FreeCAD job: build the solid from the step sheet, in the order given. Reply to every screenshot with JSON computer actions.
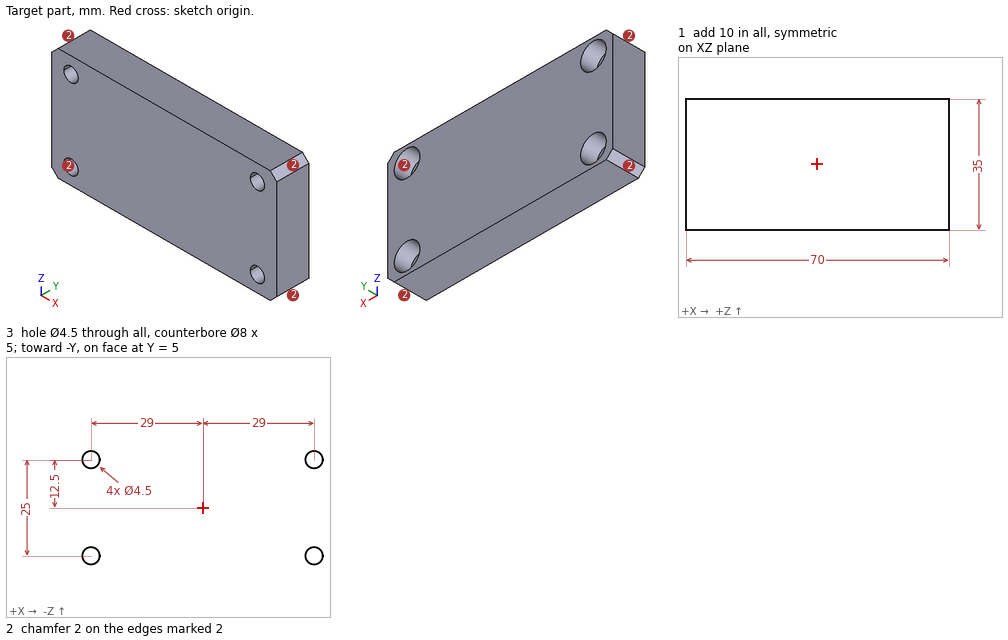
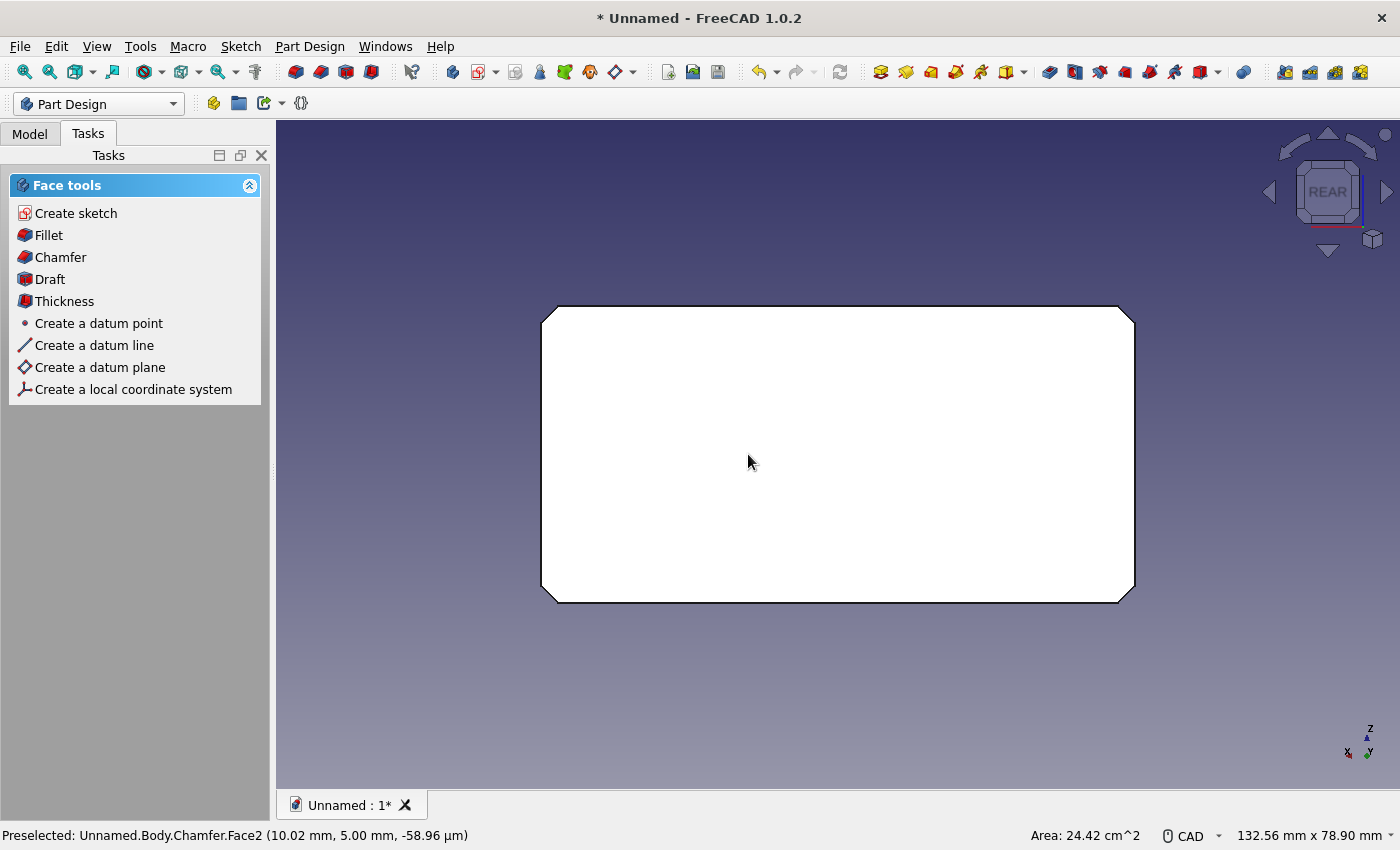
{"action": "left_click", "coordinate": [478, 72]}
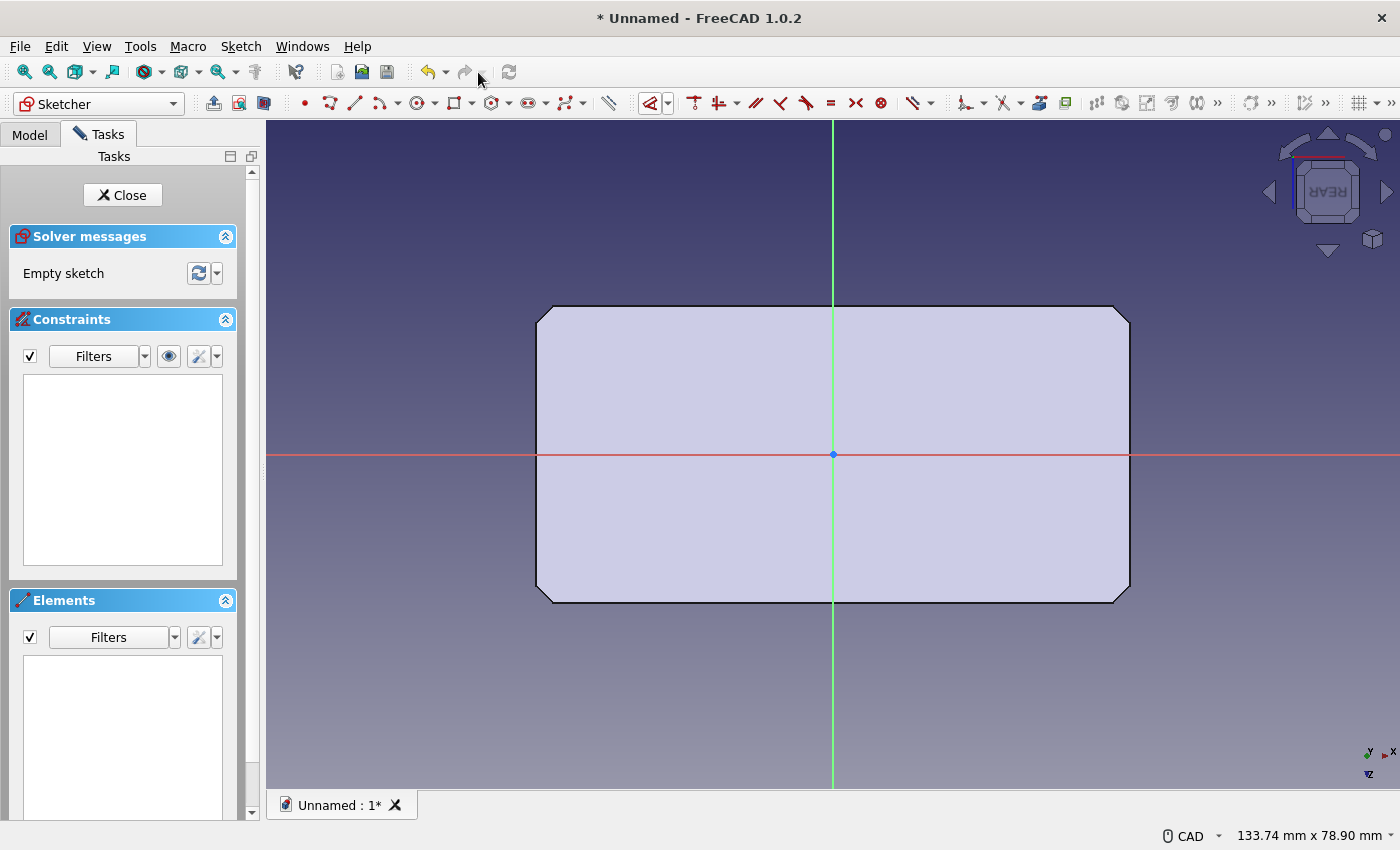
{"action": "left_click", "coordinate": [416, 104]}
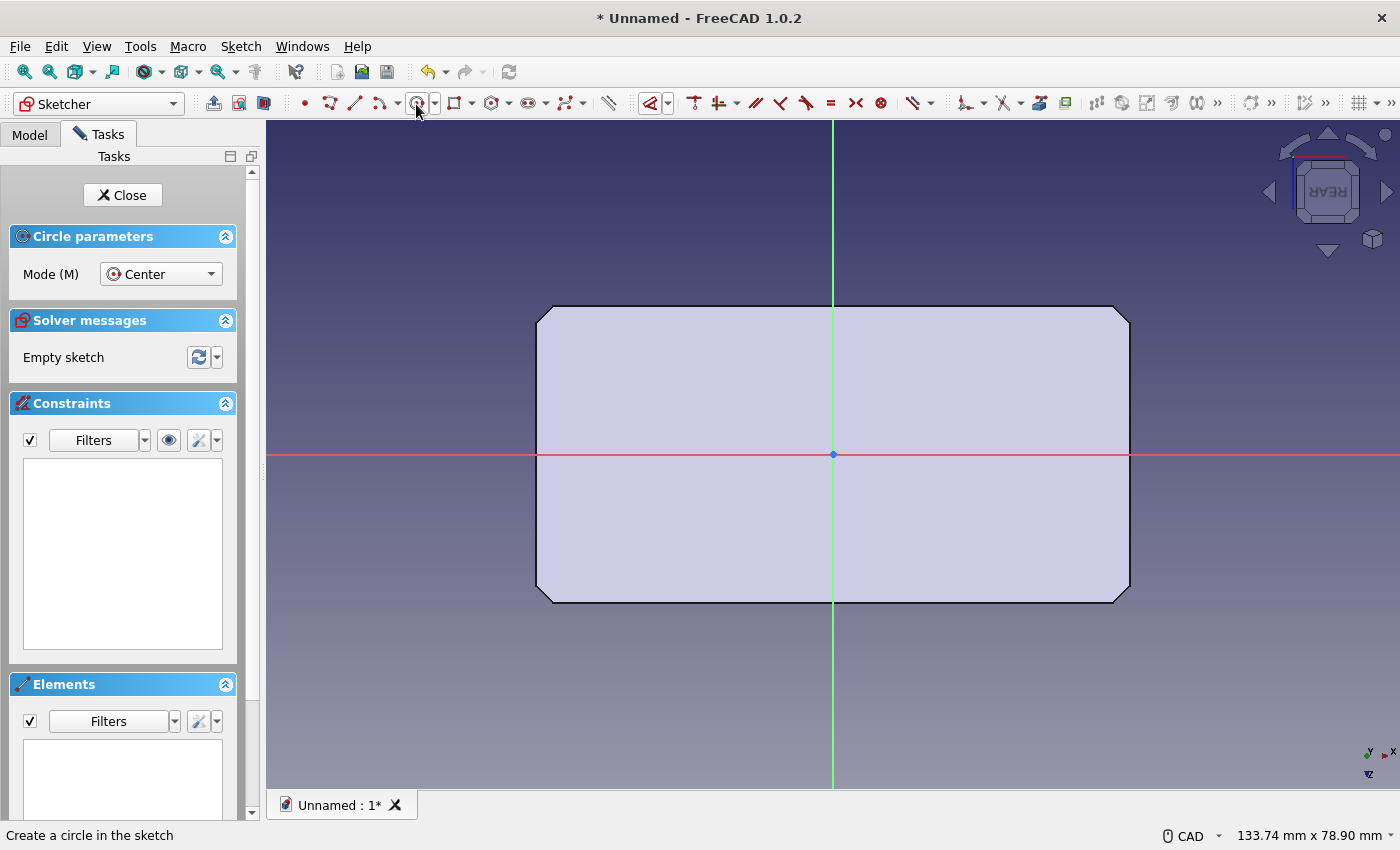
{"action": "left_click", "coordinate": [587, 349]}
{"action": "left_click", "coordinate": [601, 335]}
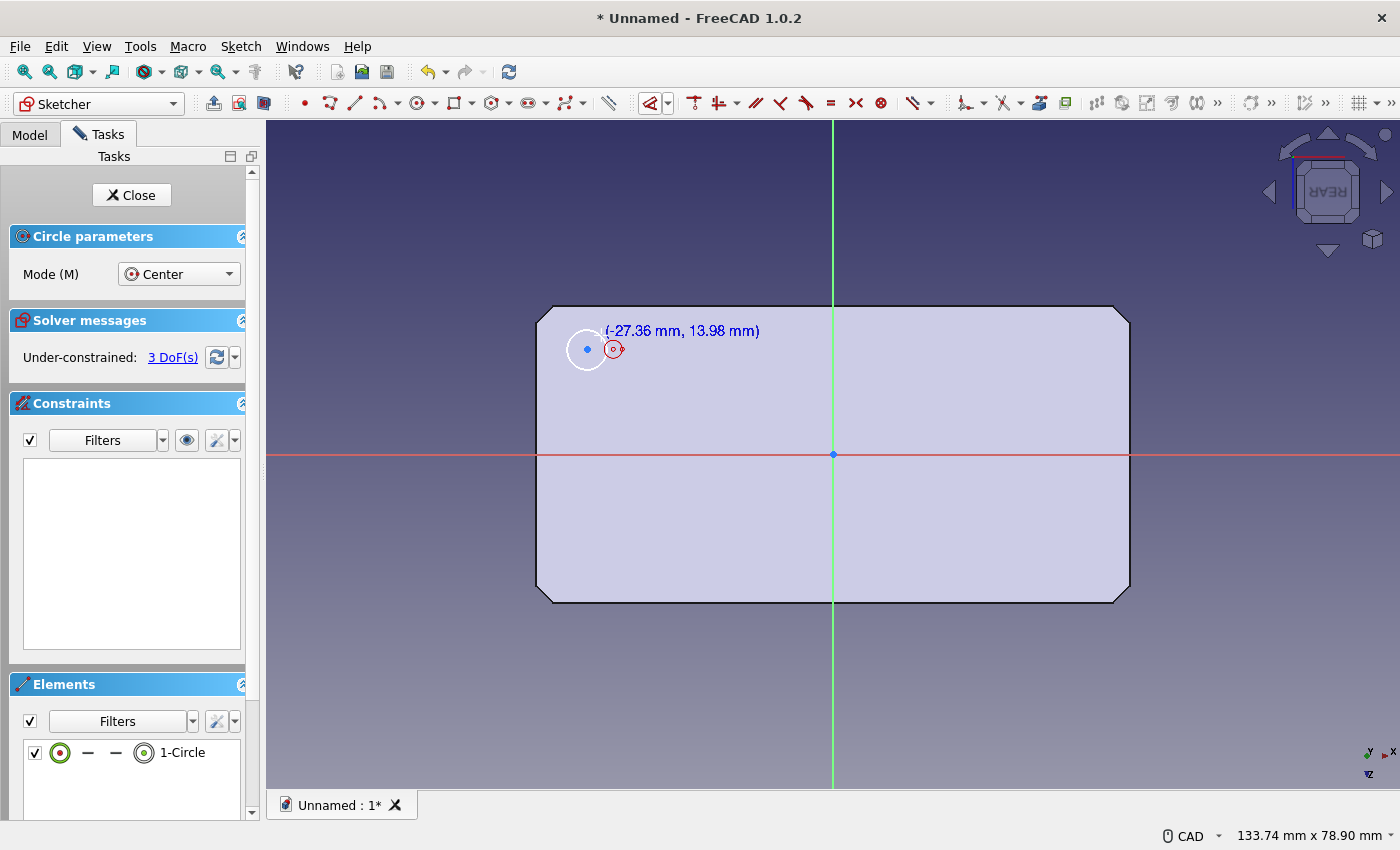
{"action": "left_click", "coordinate": [587, 560]}
{"action": "left_click", "coordinate": [601, 547]}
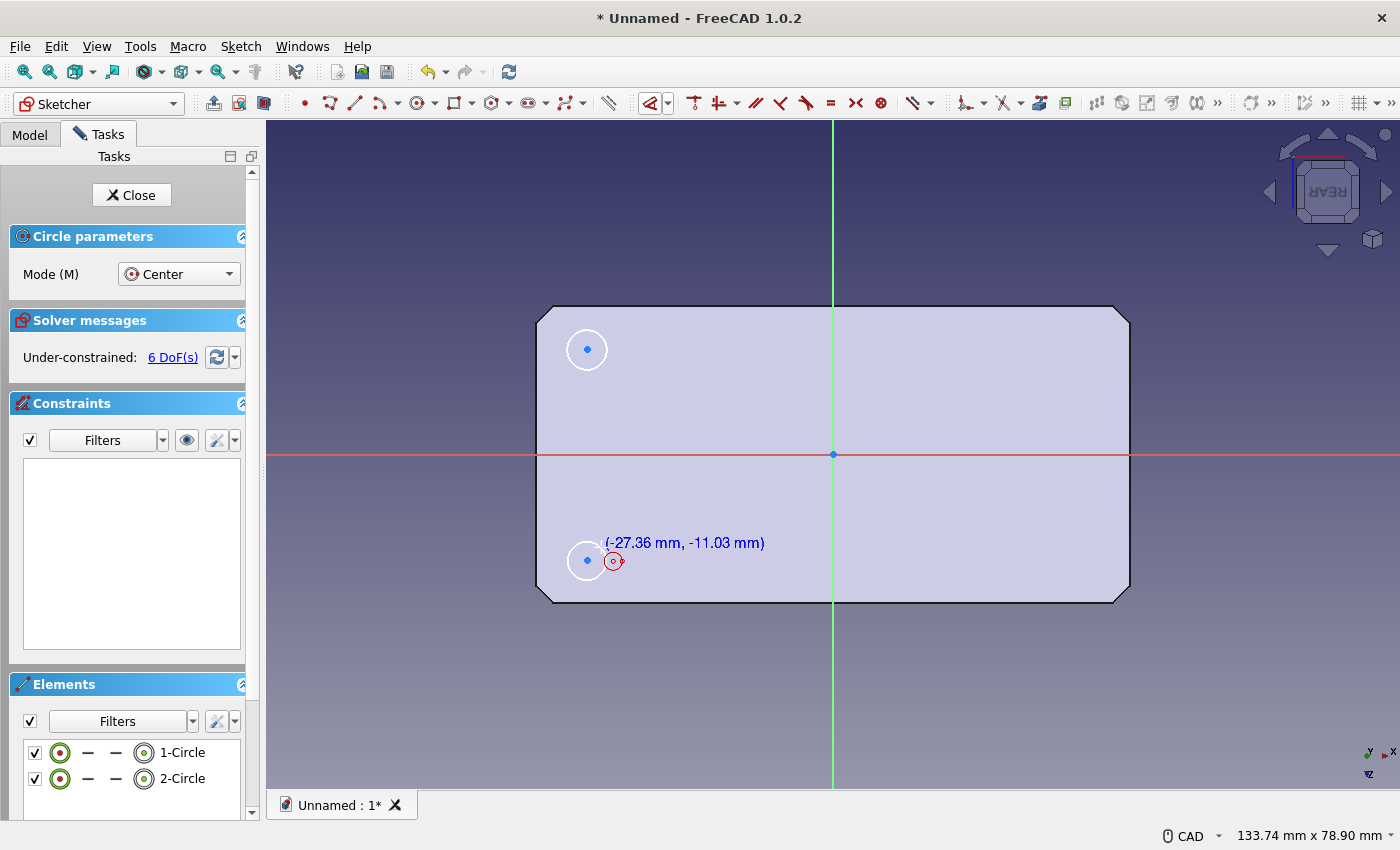
{"action": "left_click", "coordinate": [1079, 349]}
{"action": "left_click", "coordinate": [1092, 335]}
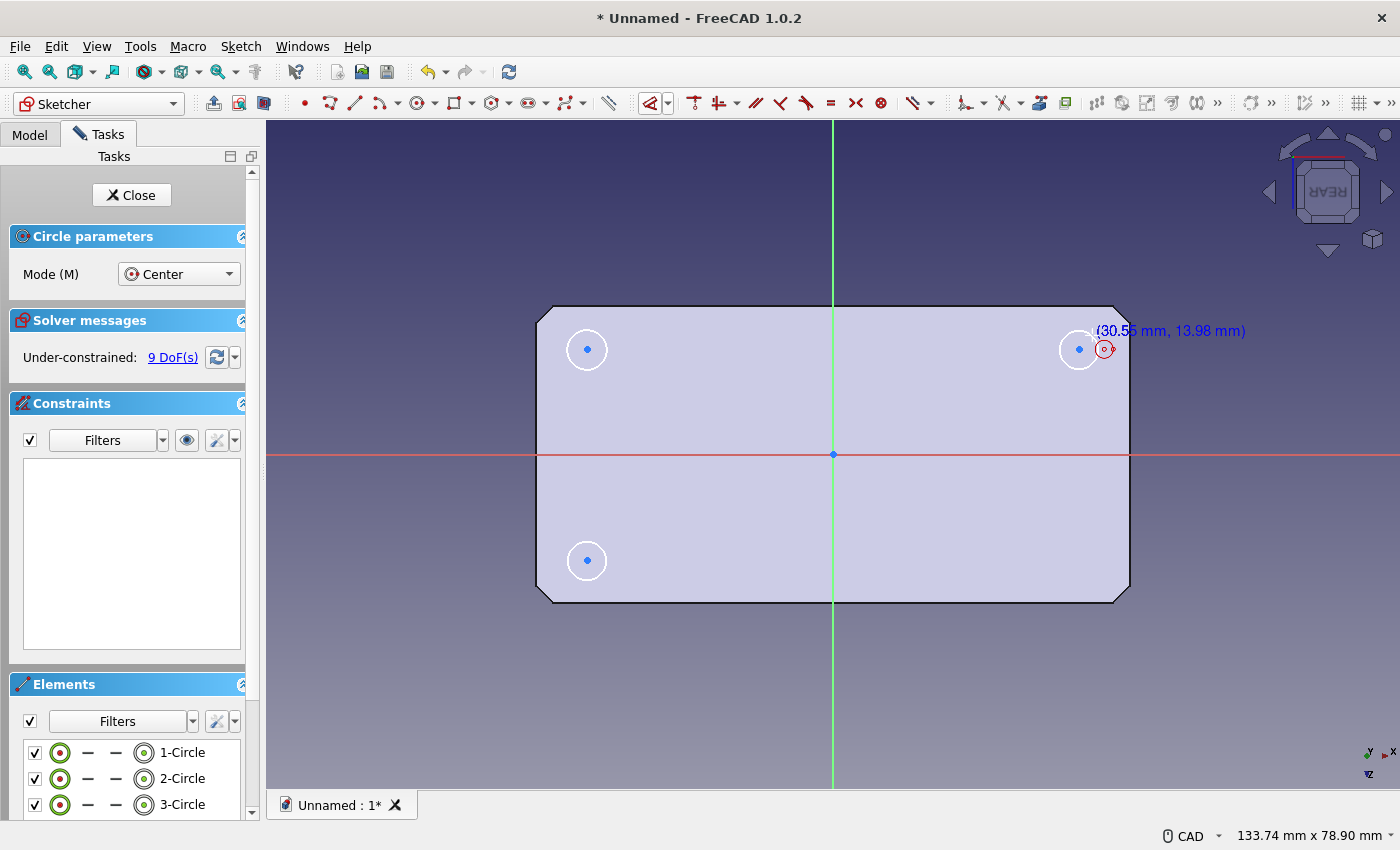
{"action": "left_click", "coordinate": [1079, 560]}
{"action": "left_click", "coordinate": [1092, 547]}
{"action": "key", "text": "Escape"}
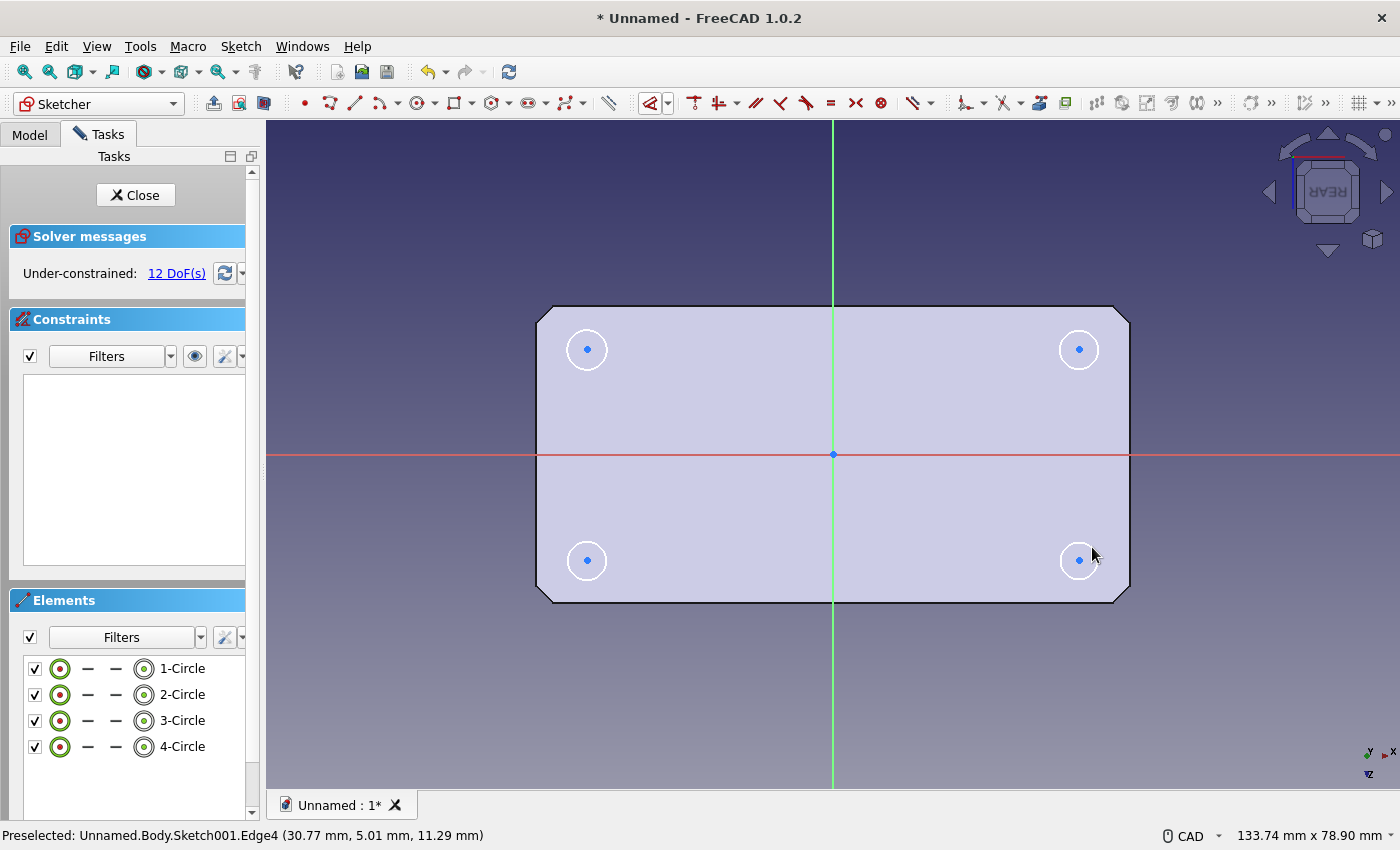
{"action": "left_click", "coordinate": [601, 336]}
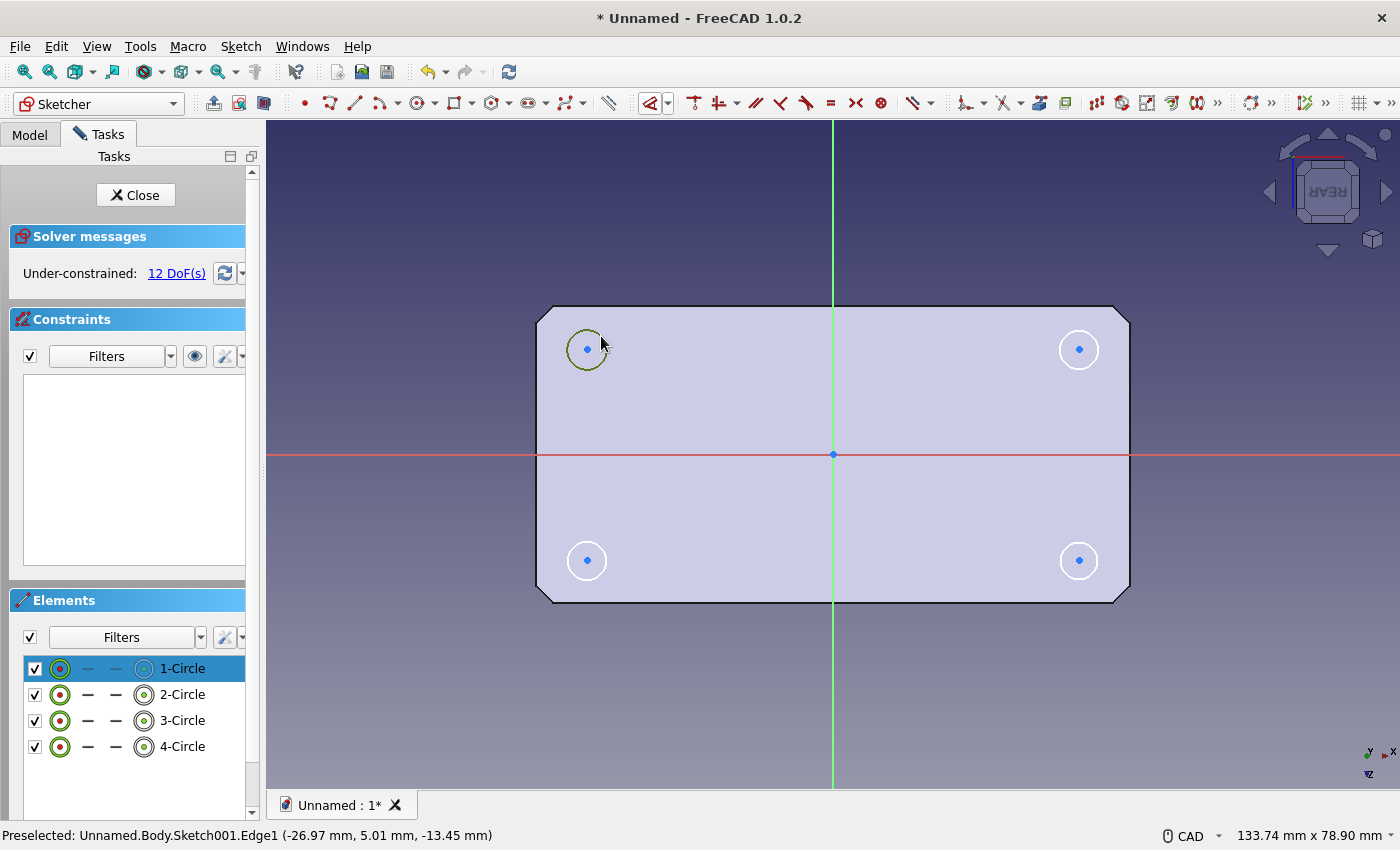
{"action": "left_click", "coordinate": [600, 547]}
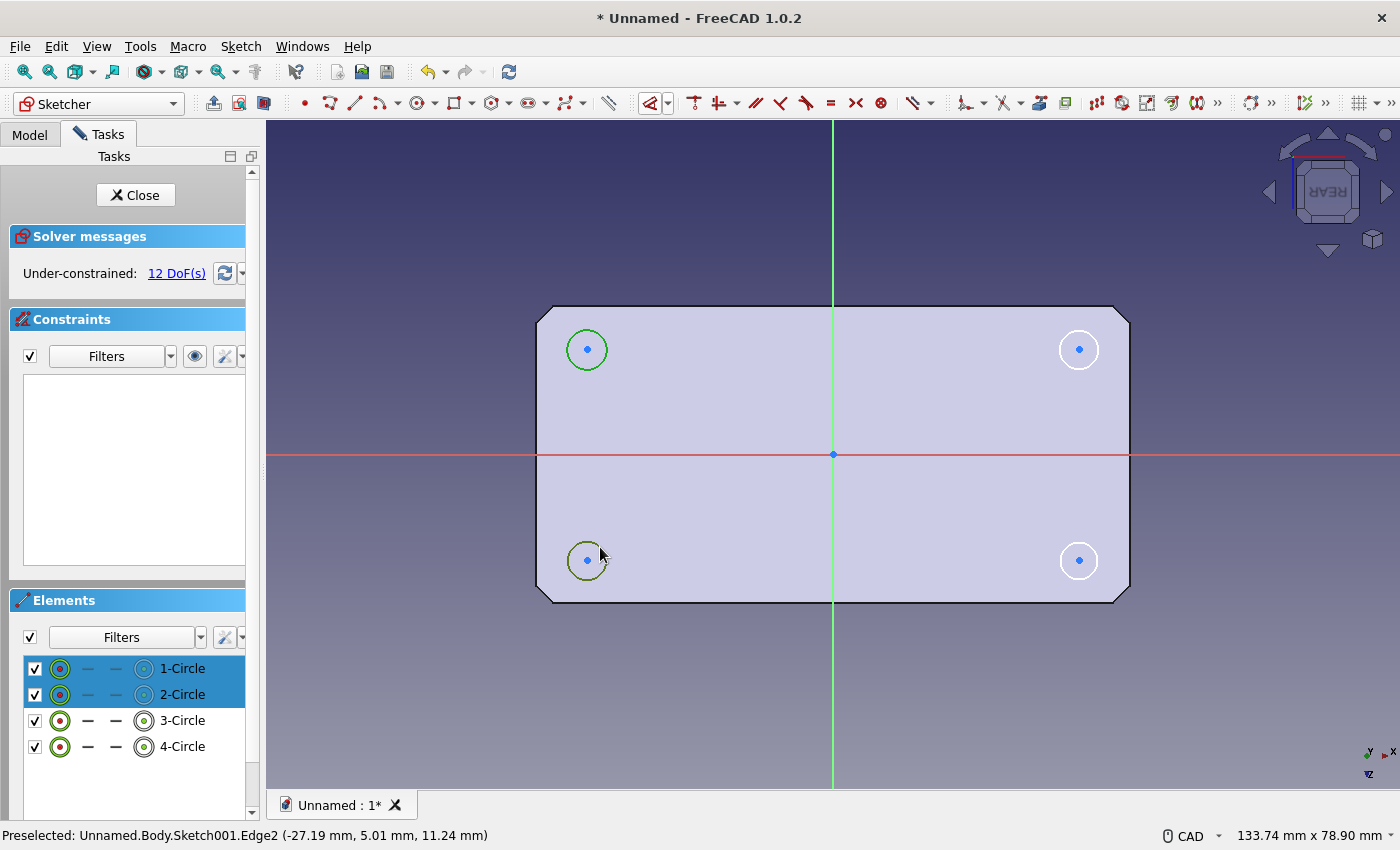
{"action": "left_click", "coordinate": [1092, 336]}